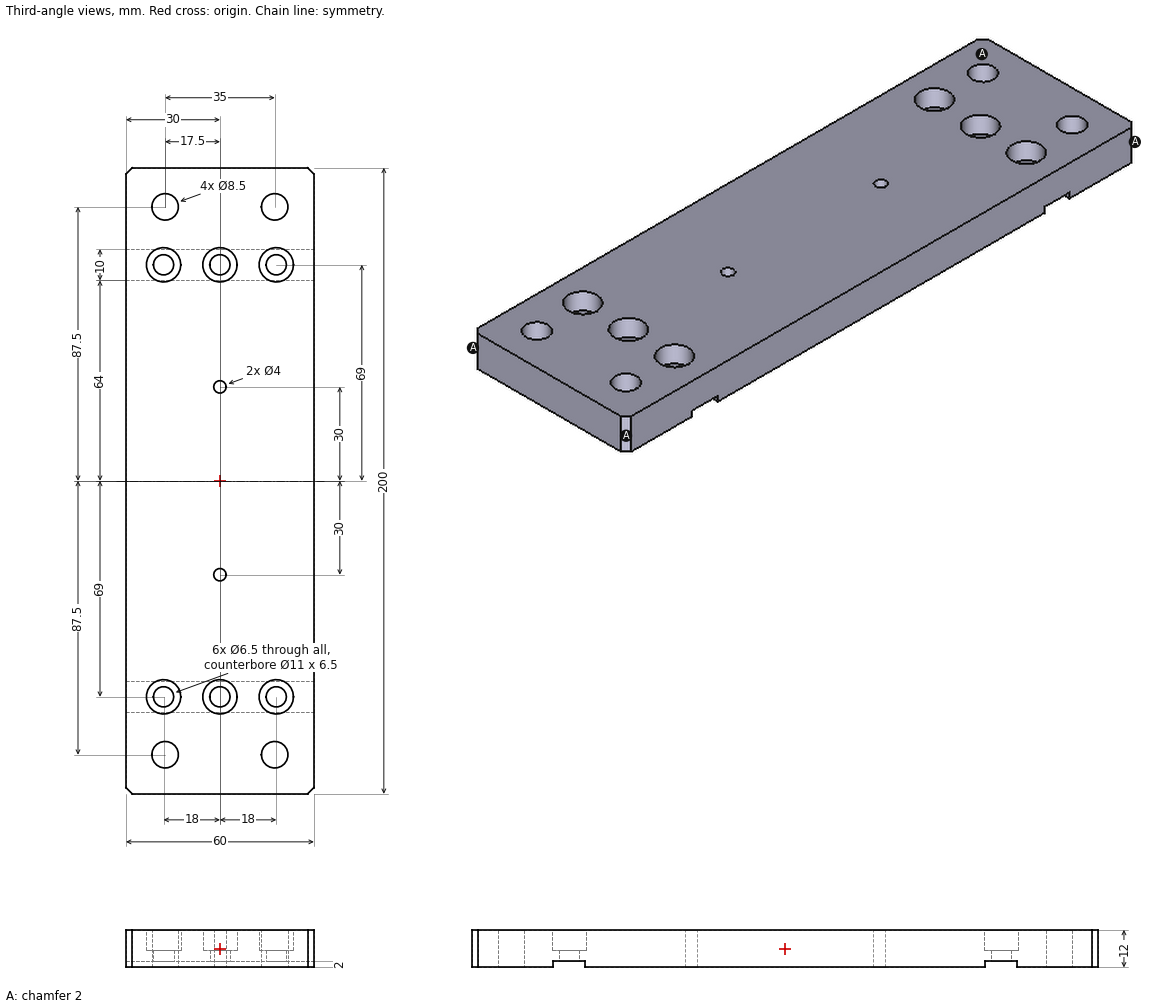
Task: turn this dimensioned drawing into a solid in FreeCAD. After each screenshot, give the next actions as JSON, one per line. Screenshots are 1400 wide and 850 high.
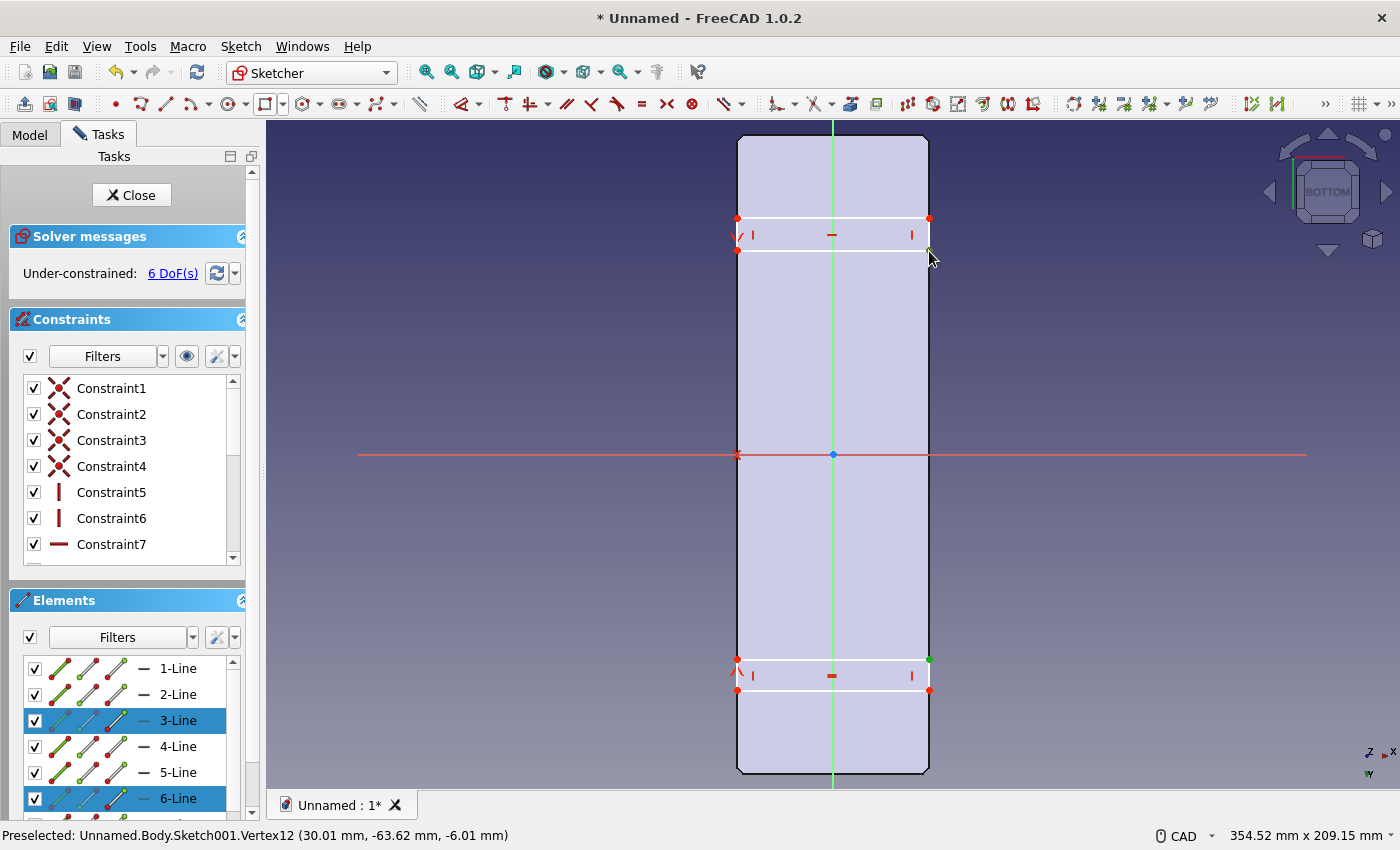
{"action": "left_click", "coordinate": [361, 454]}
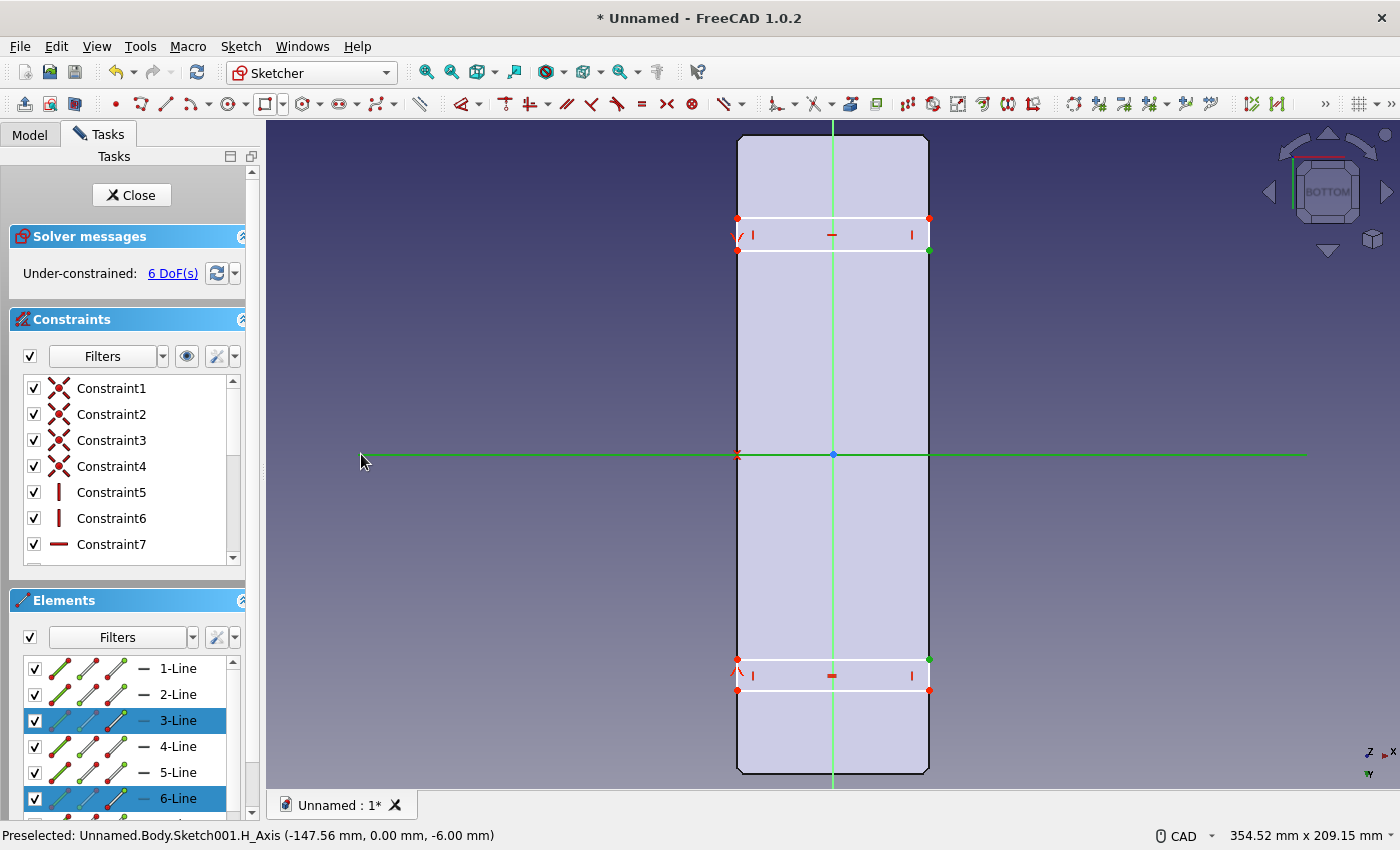
{"action": "left_click", "coordinate": [667, 104]}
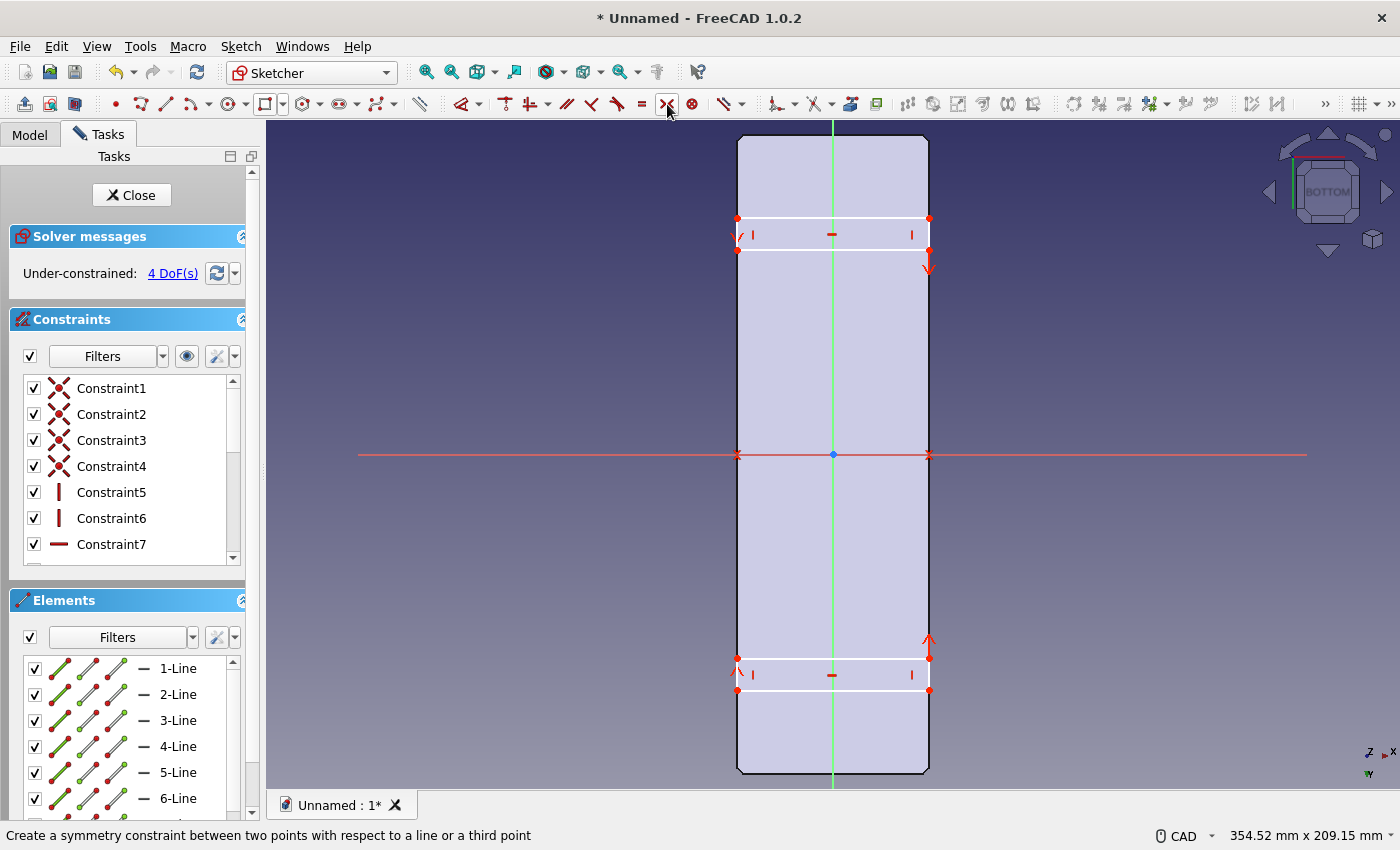
{"action": "left_click", "coordinate": [460, 104]}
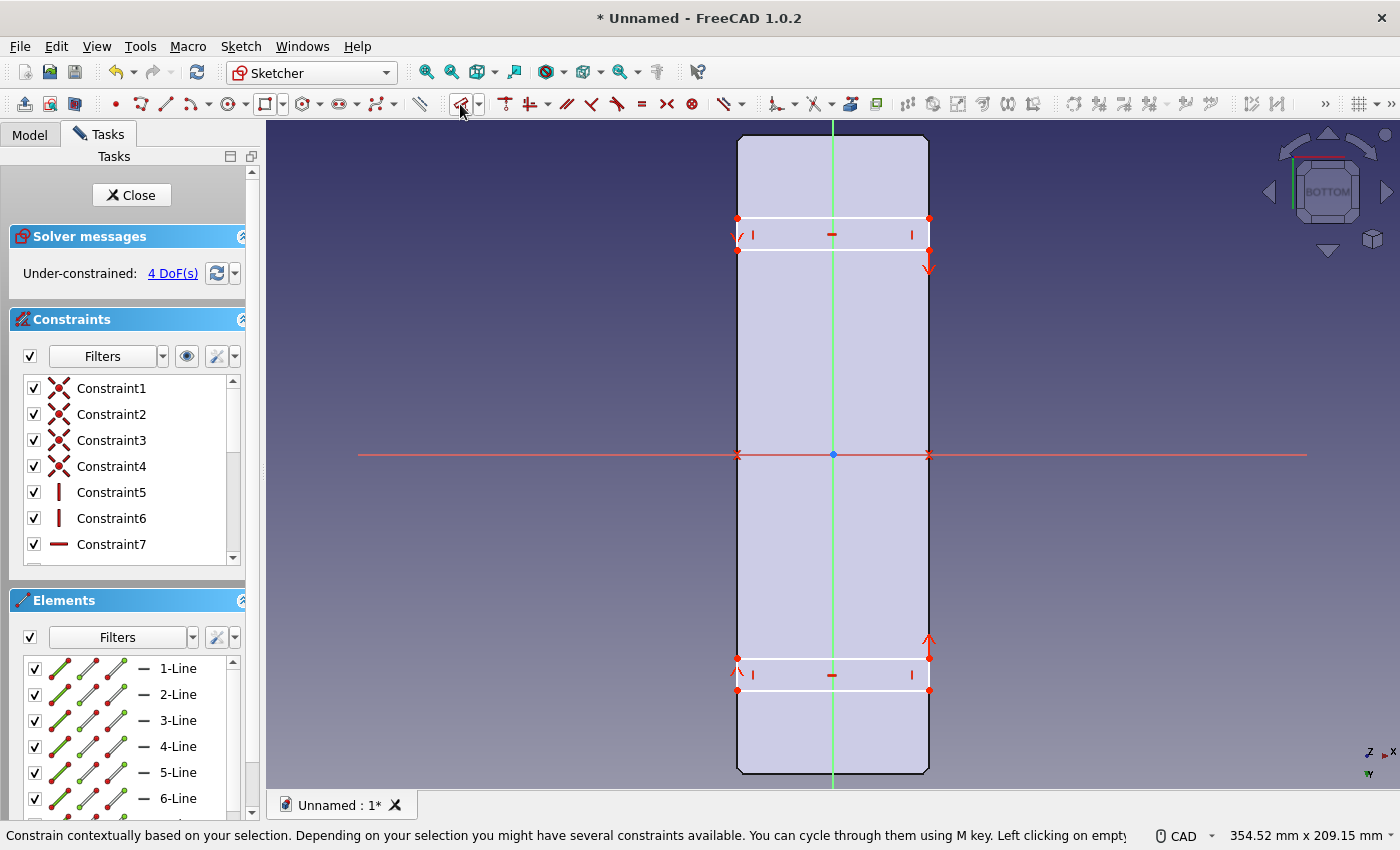
{"action": "scroll", "coordinate": [737, 669], "scroll_direction": "up", "scroll_amount": 2}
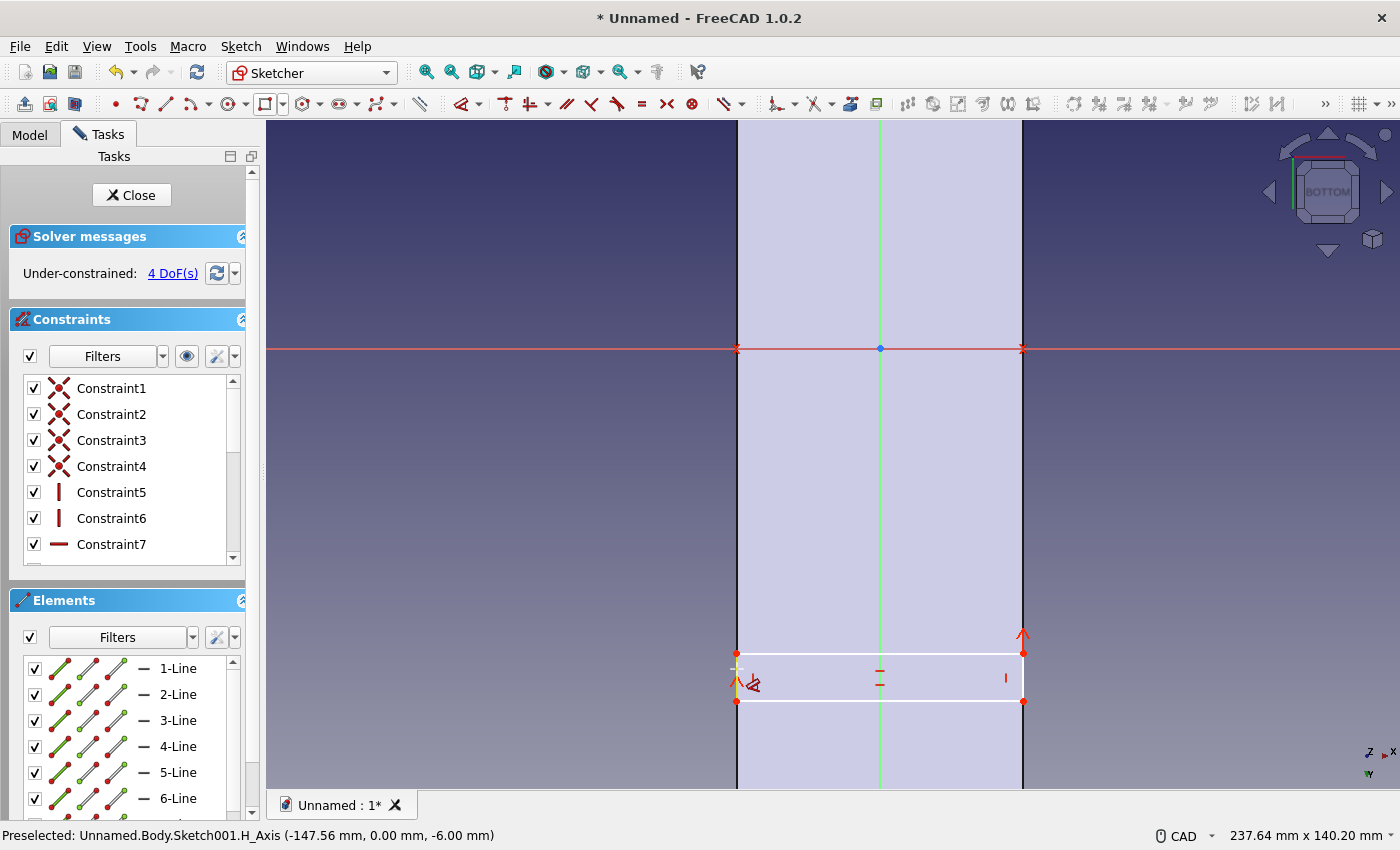
{"action": "left_click", "coordinate": [737, 668]}
{"action": "left_click", "coordinate": [703, 677]}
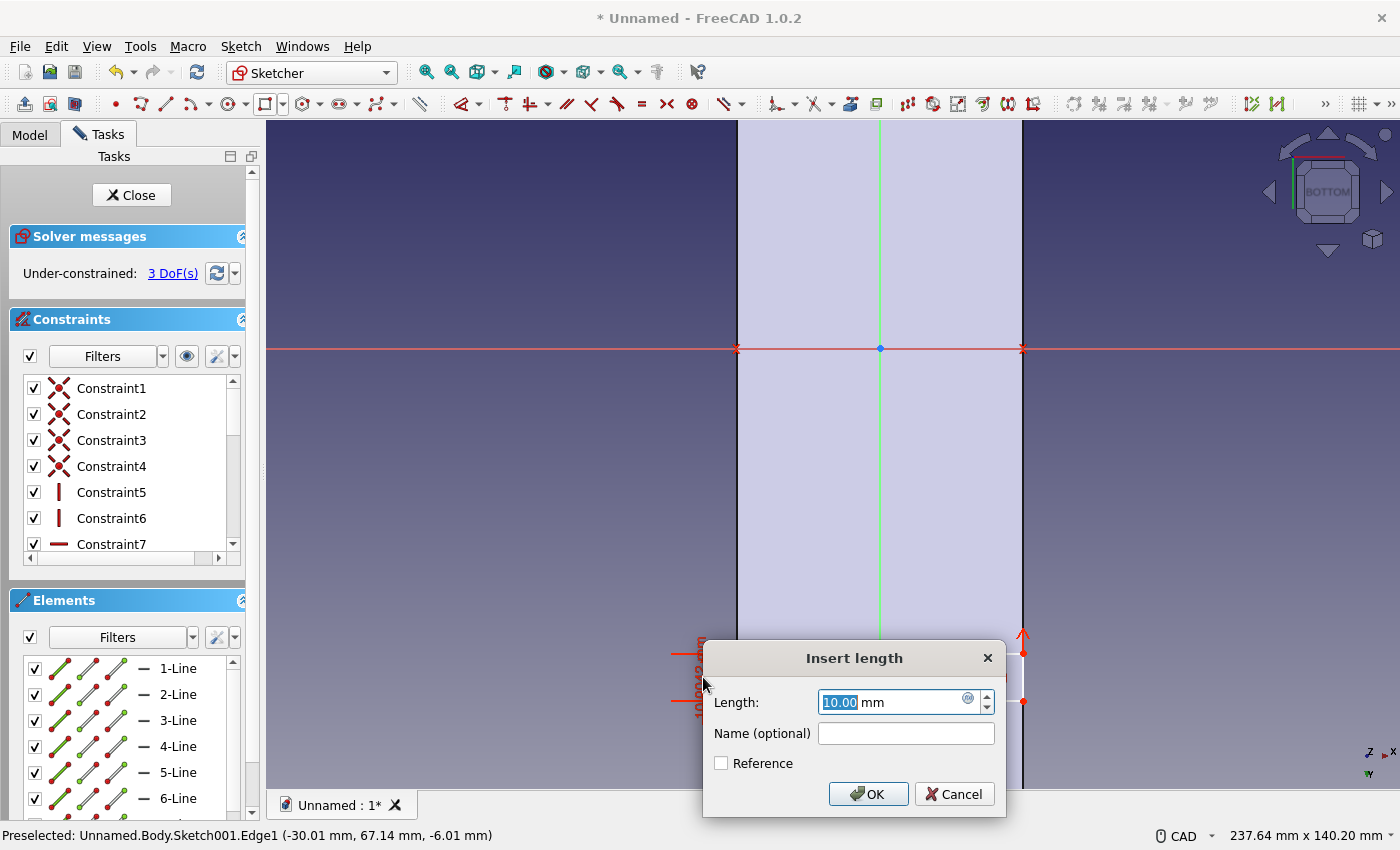
{"action": "type", "text": "10"}
{"action": "key", "text": "Return"}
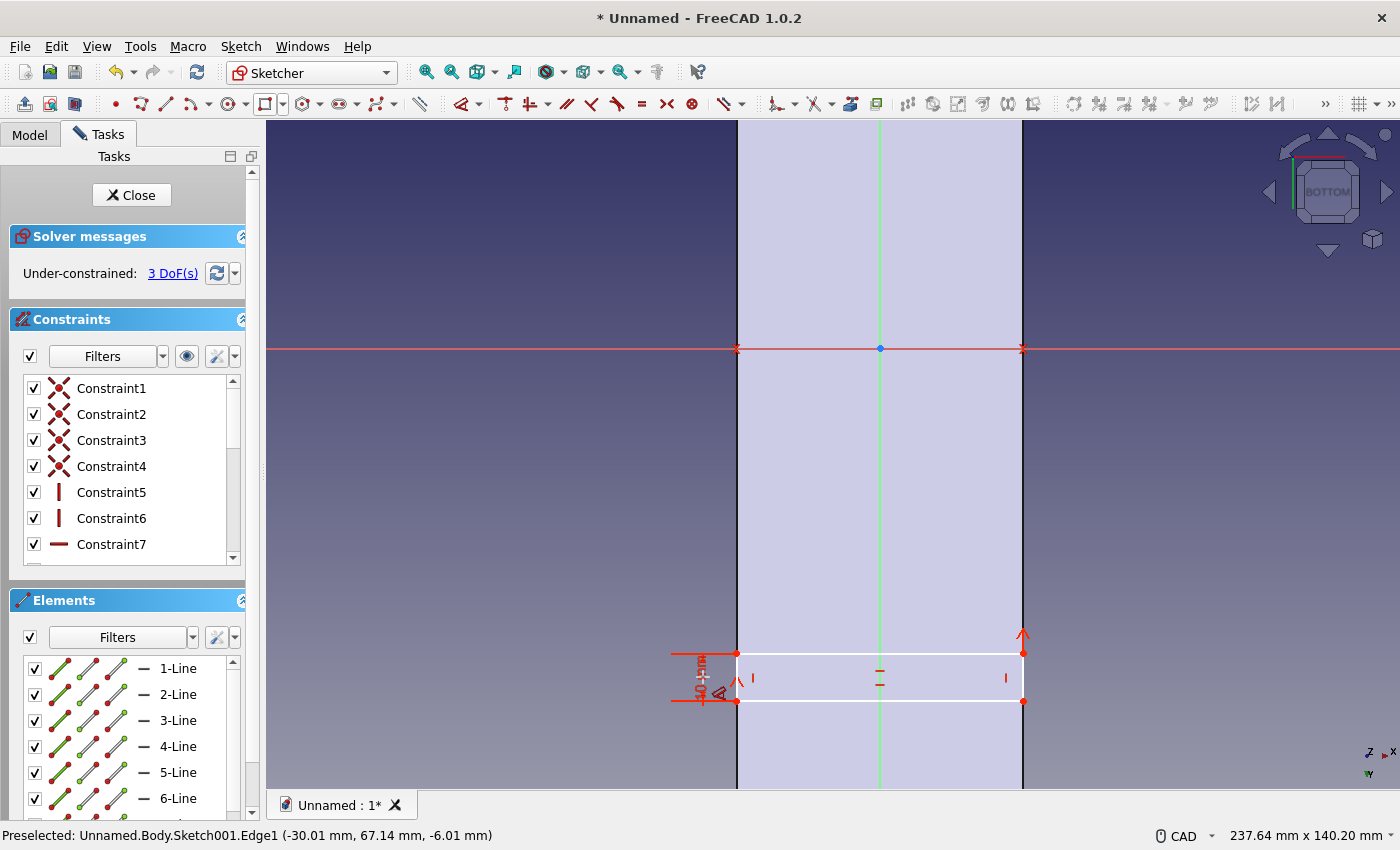
{"action": "left_click", "coordinate": [823, 701]}
{"action": "left_click", "coordinate": [814, 735]}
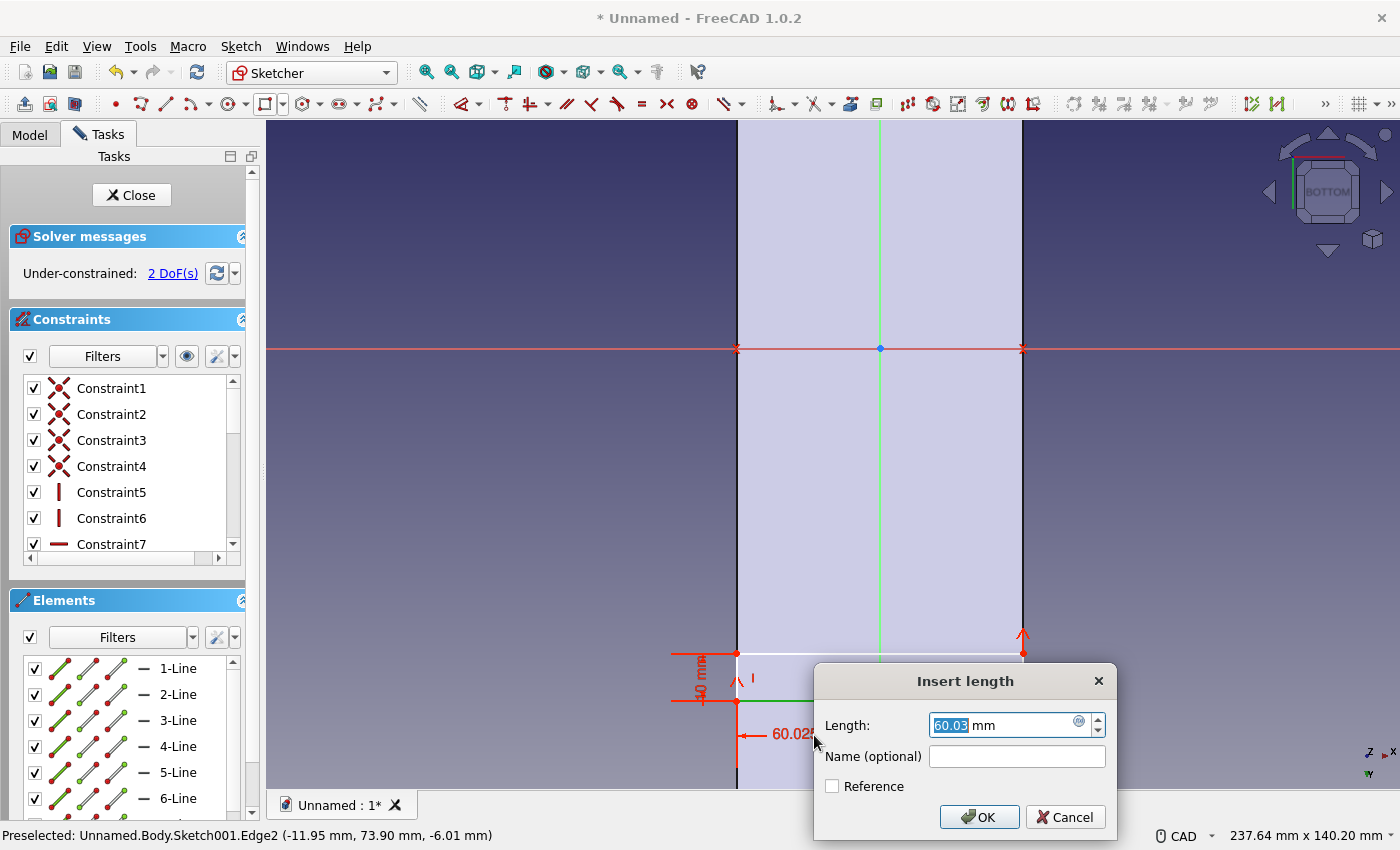
{"action": "type", "text": "60"}
{"action": "key", "text": "Return"}